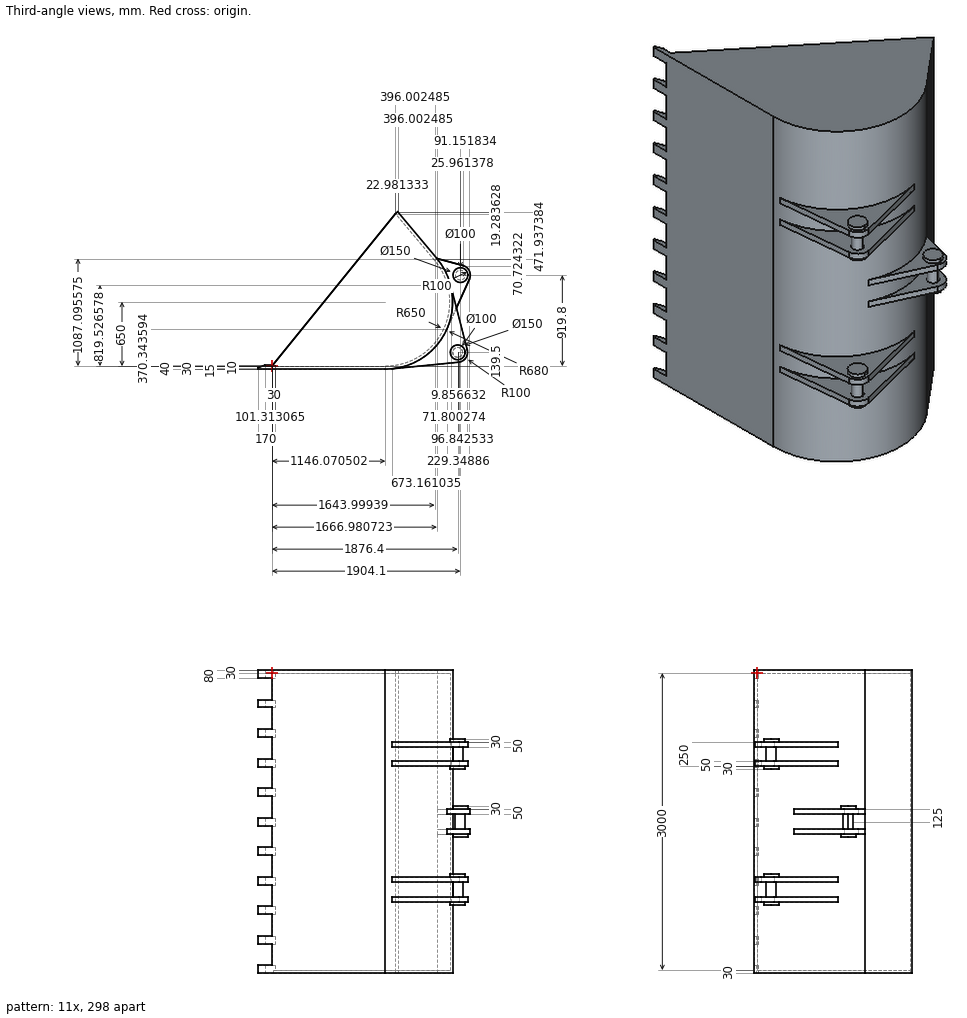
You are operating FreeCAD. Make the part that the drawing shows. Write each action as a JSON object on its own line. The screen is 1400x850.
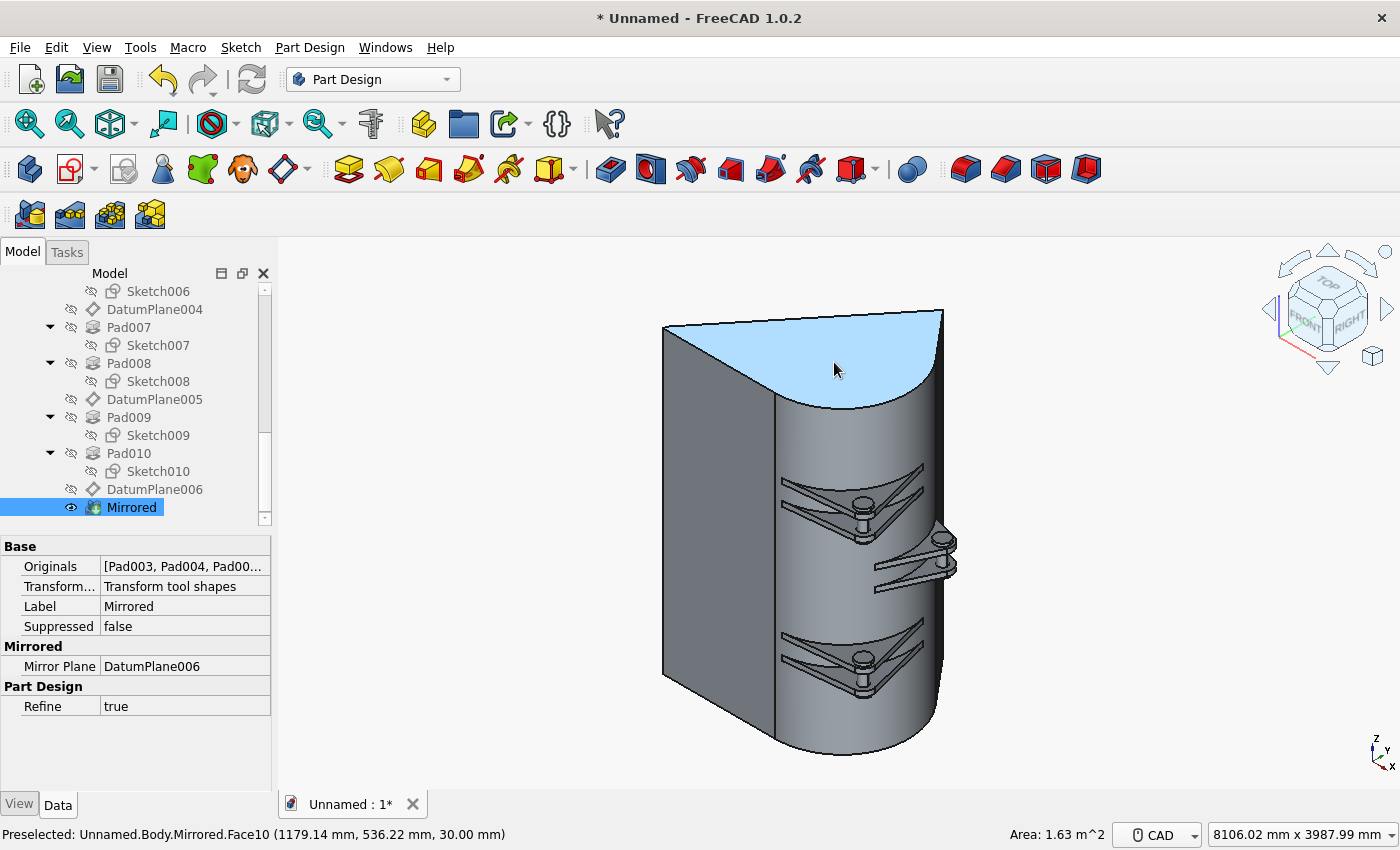
{"action": "left_click", "coordinate": [70, 170]}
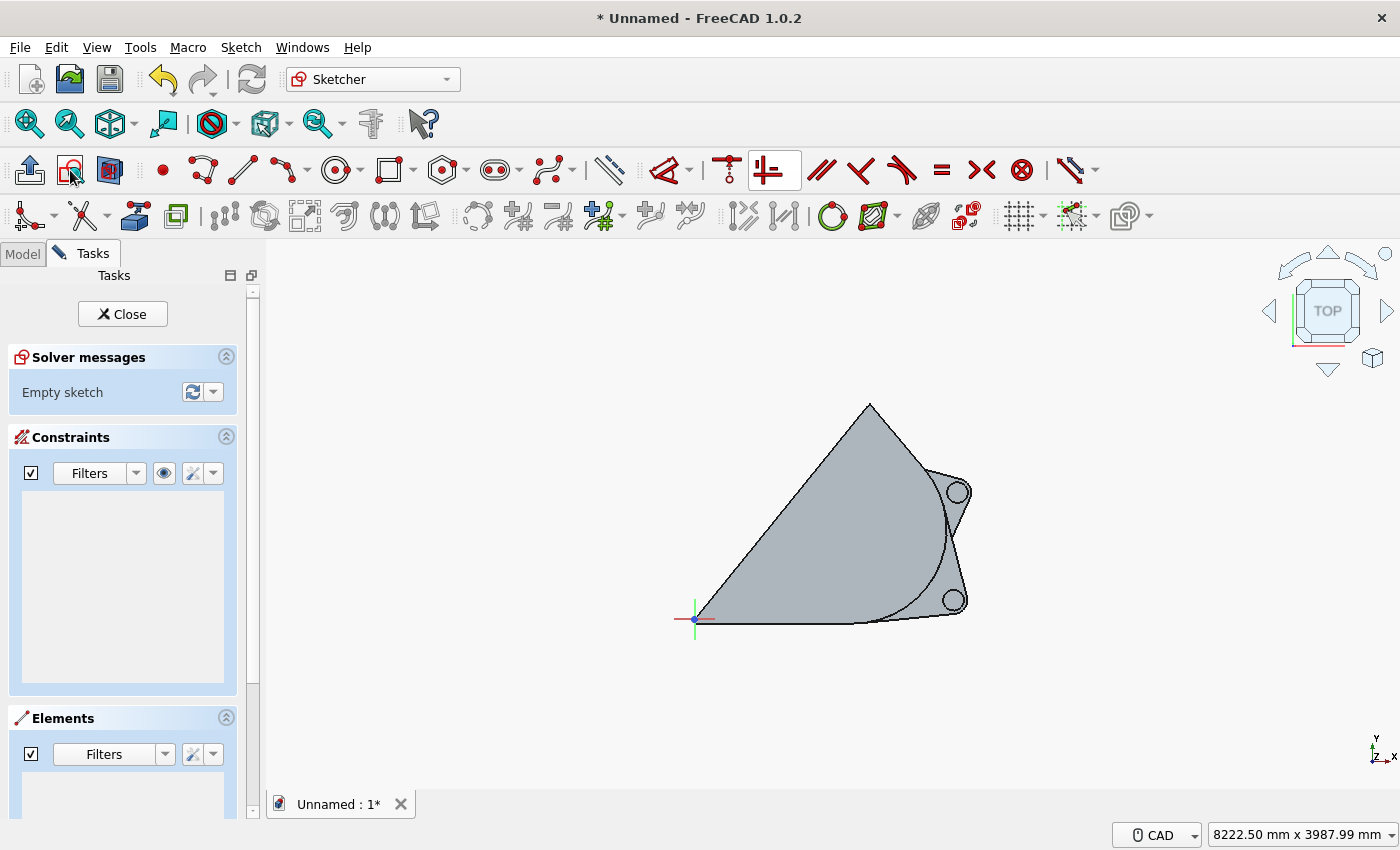
{"action": "scroll", "coordinate": [683, 626], "scroll_direction": "up", "scroll_amount": 15}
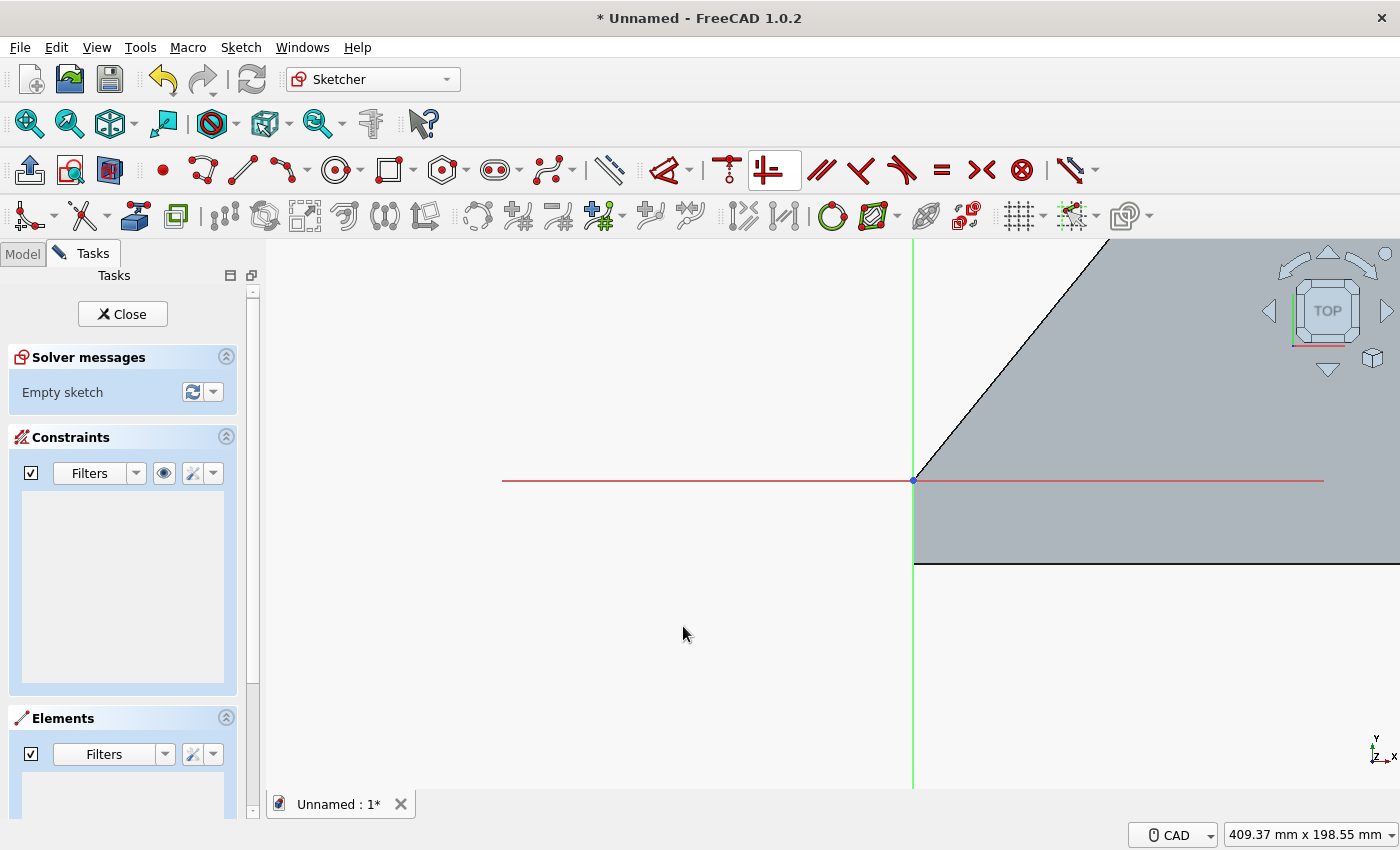
{"action": "scroll", "coordinate": [754, 497], "scroll_direction": "up", "scroll_amount": 2}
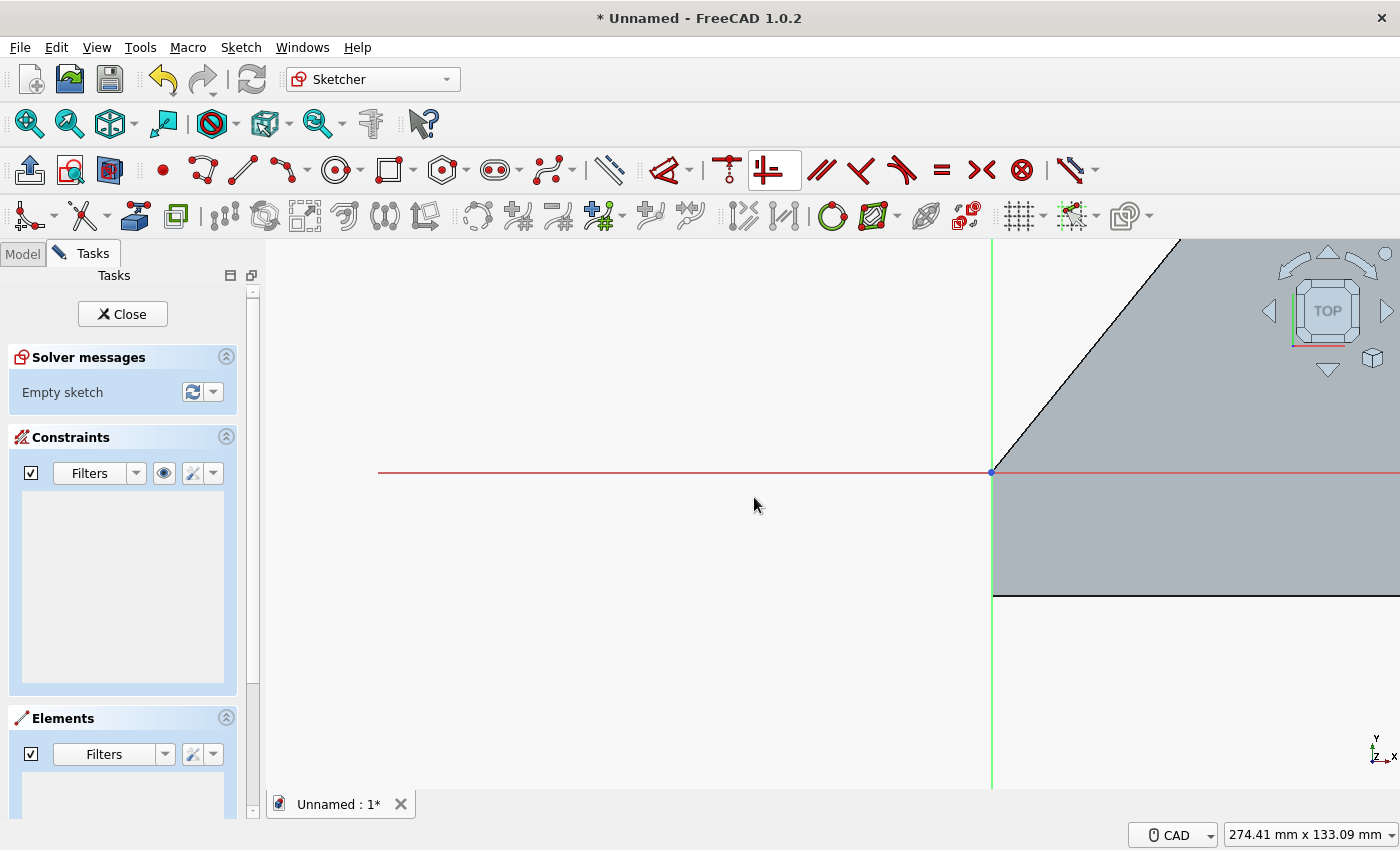
{"action": "left_click", "coordinate": [204, 170]}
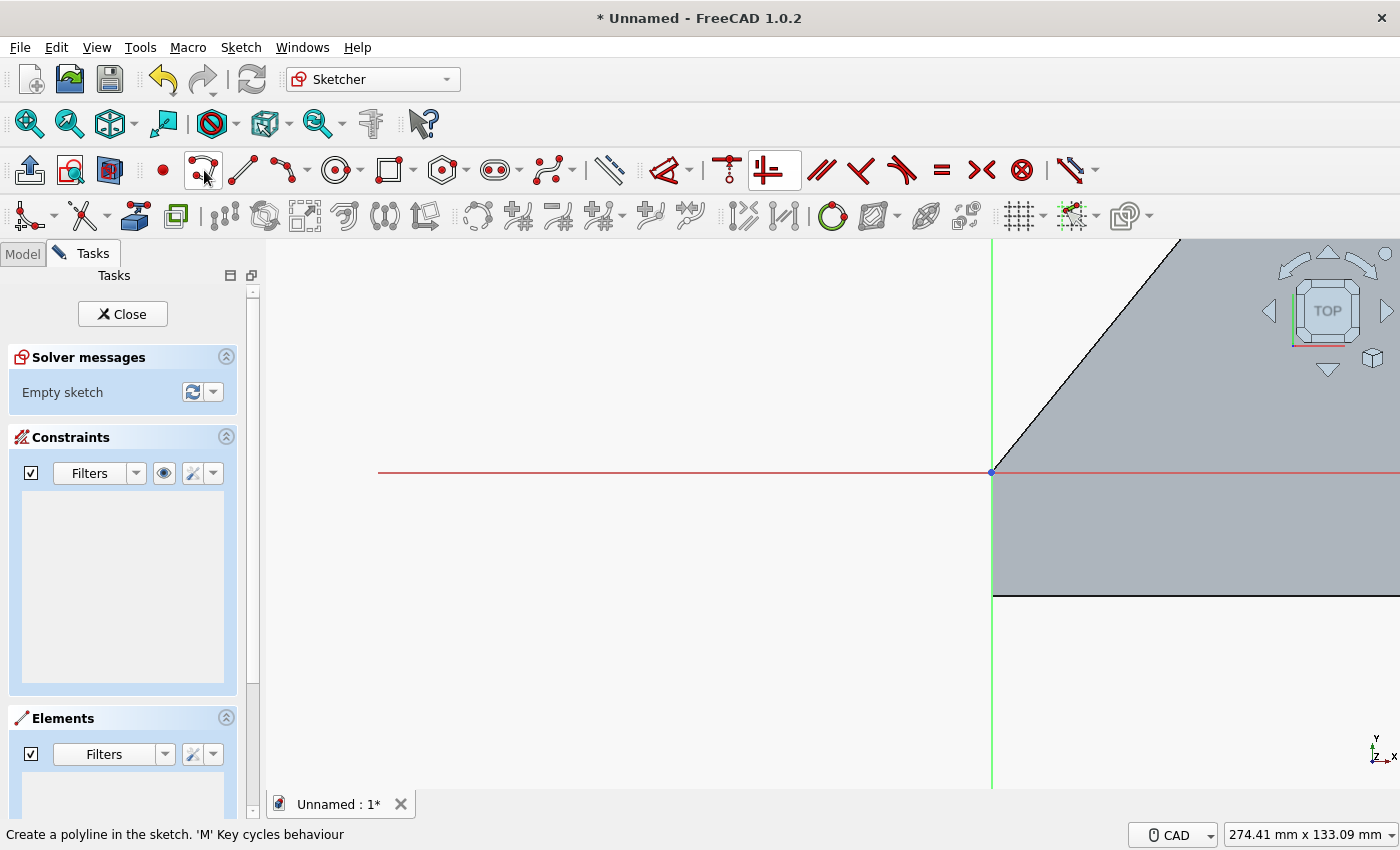
{"action": "left_click", "coordinate": [1116, 431]}
{"action": "left_click", "coordinate": [697, 431]}
{"action": "left_click", "coordinate": [413, 534]}
{"action": "left_click", "coordinate": [413, 596]}
{"action": "left_click", "coordinate": [1116, 596]}
{"action": "left_click", "coordinate": [1116, 432]}
{"action": "key", "text": "Escape"}
{"action": "key", "text": "Escape"}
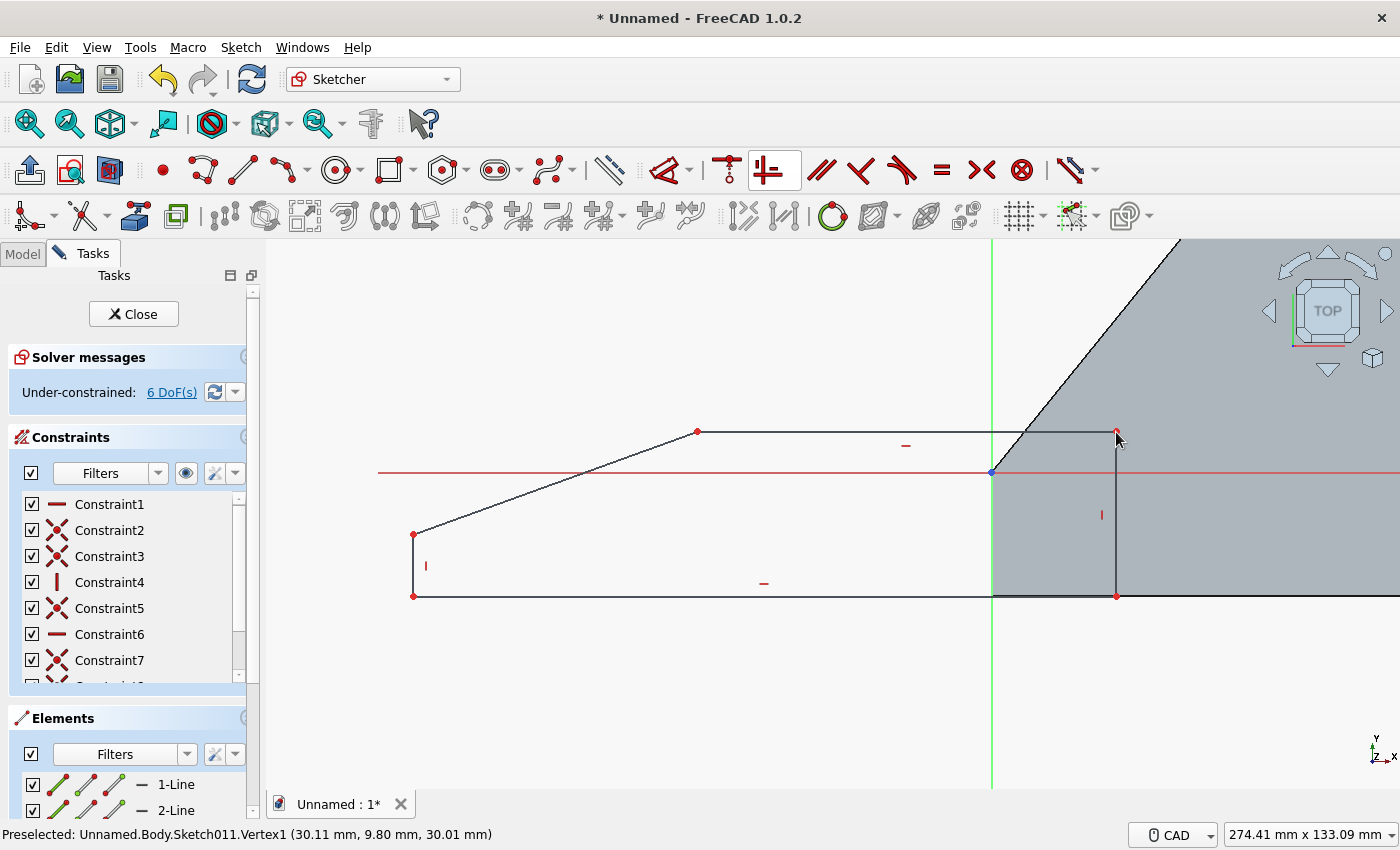
{"action": "left_click", "coordinate": [664, 170]}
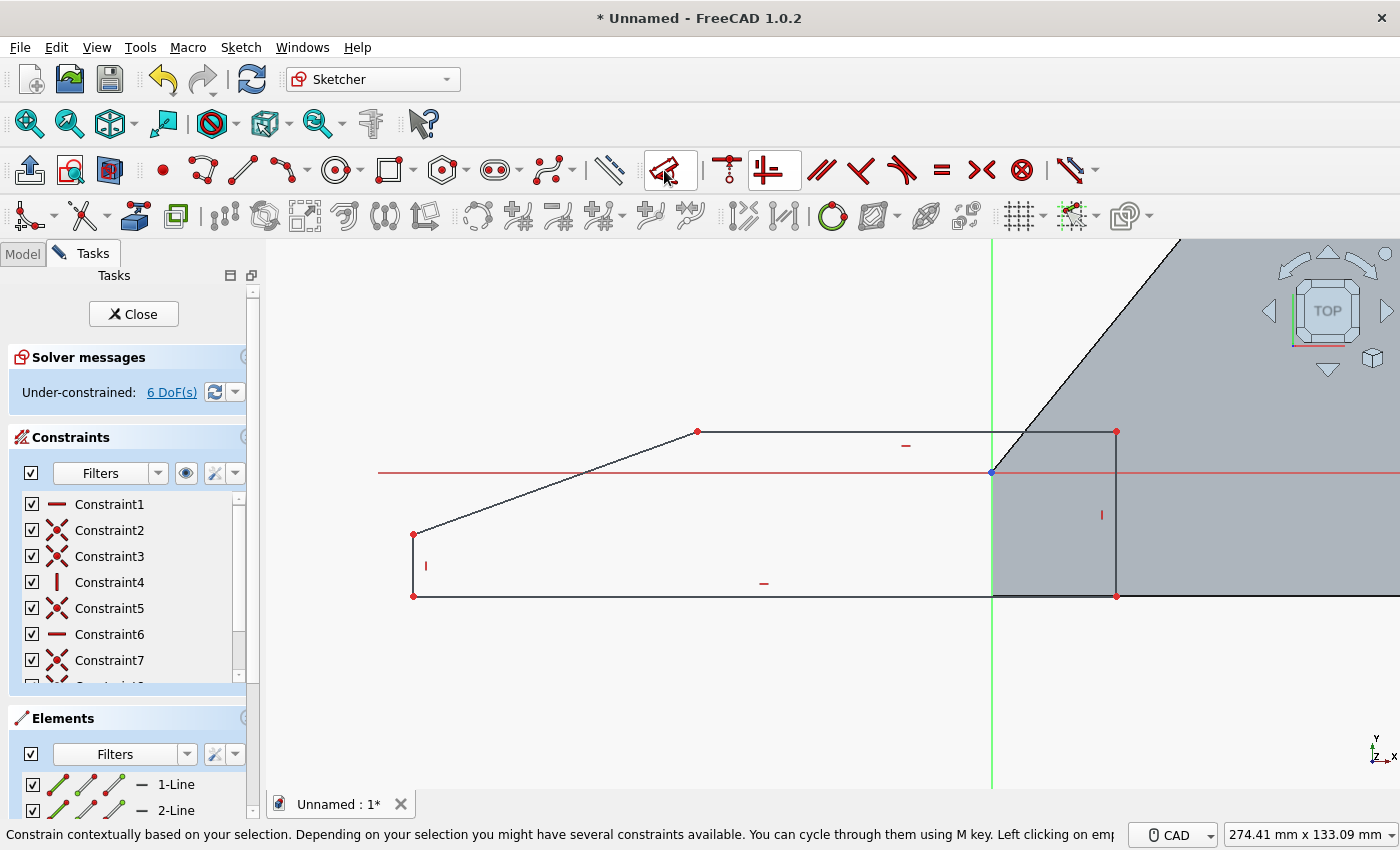
{"action": "left_click", "coordinate": [413, 554]}
{"action": "left_click", "coordinate": [379, 566]}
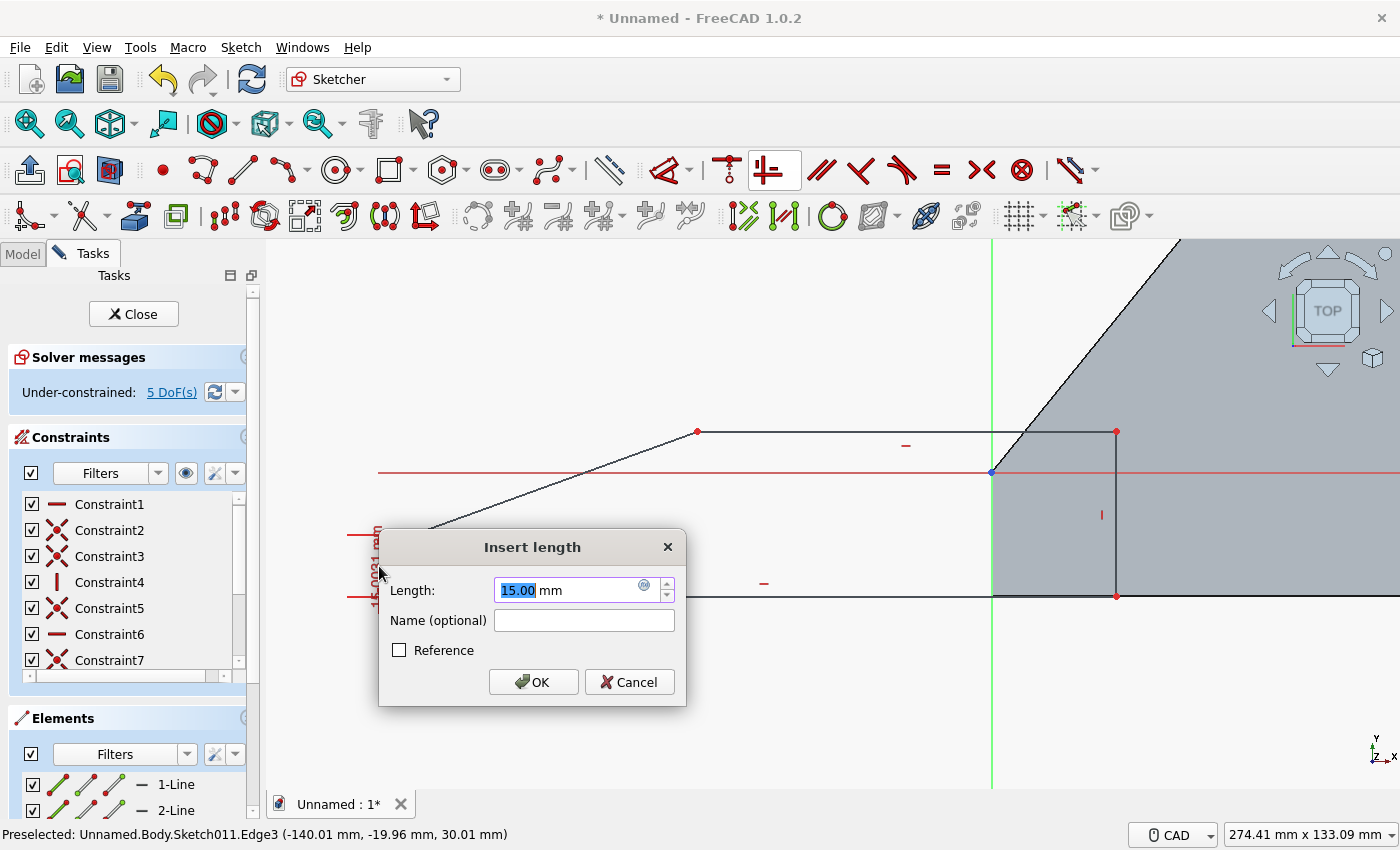
{"action": "type", "text": "15"}
{"action": "key", "text": "Return"}